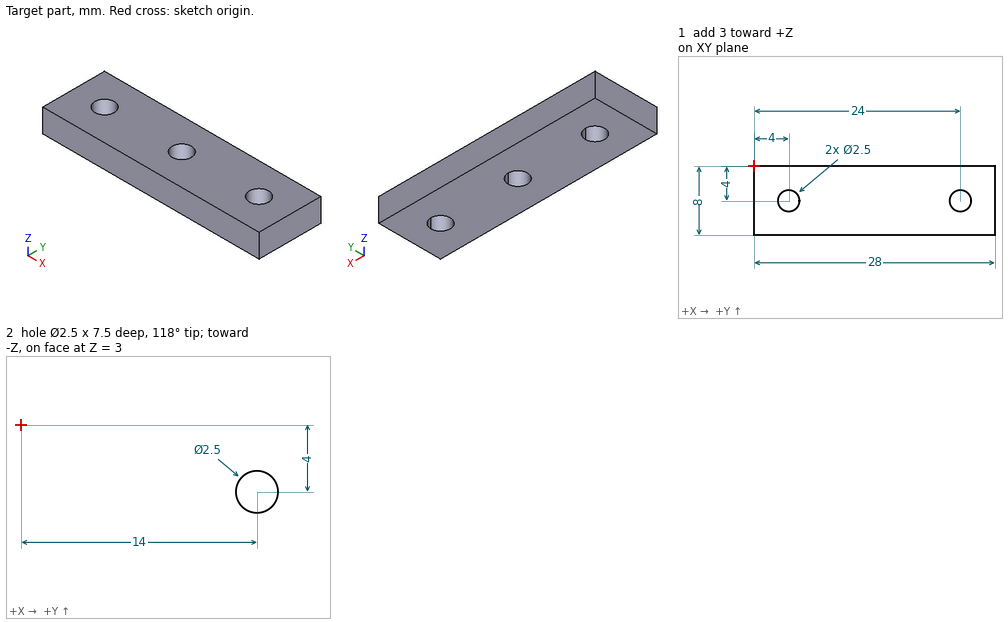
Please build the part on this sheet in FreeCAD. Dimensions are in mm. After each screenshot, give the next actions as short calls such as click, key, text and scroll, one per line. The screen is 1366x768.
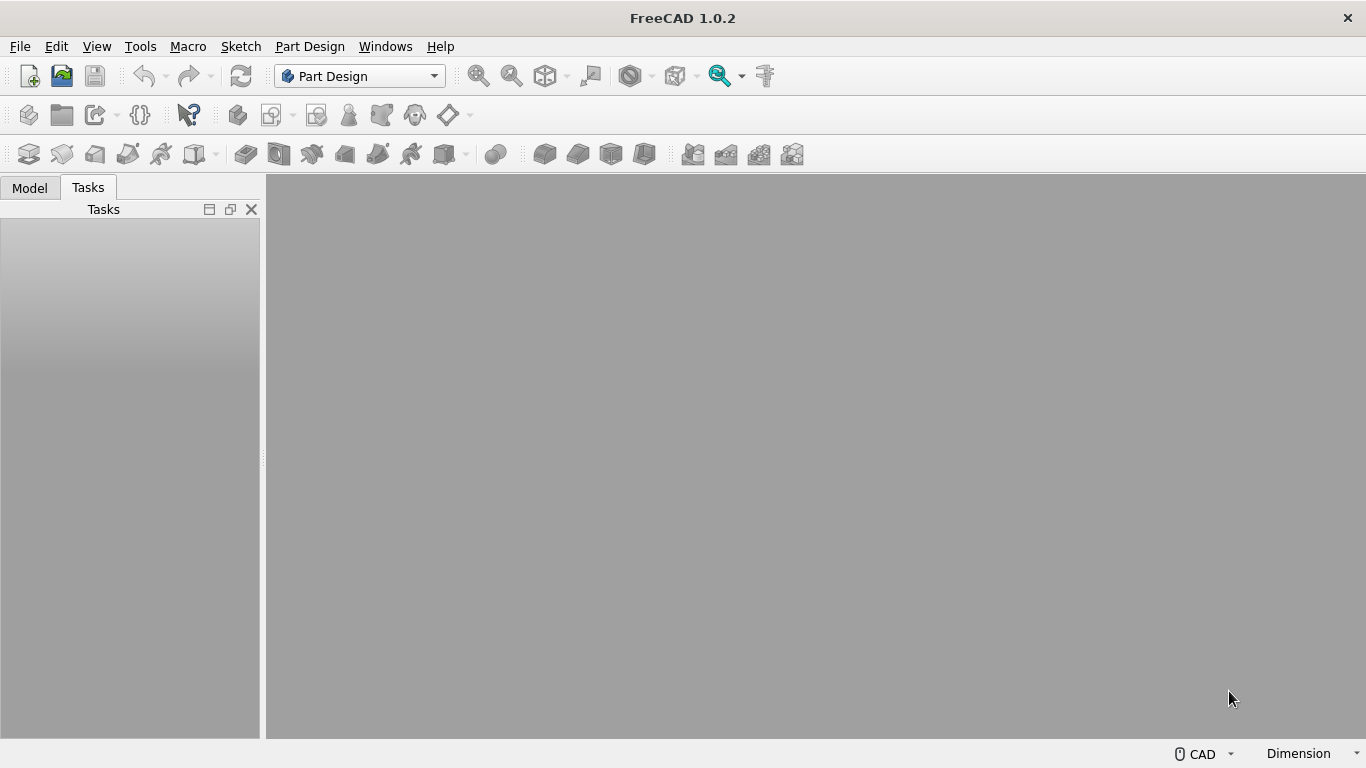
click(29, 76)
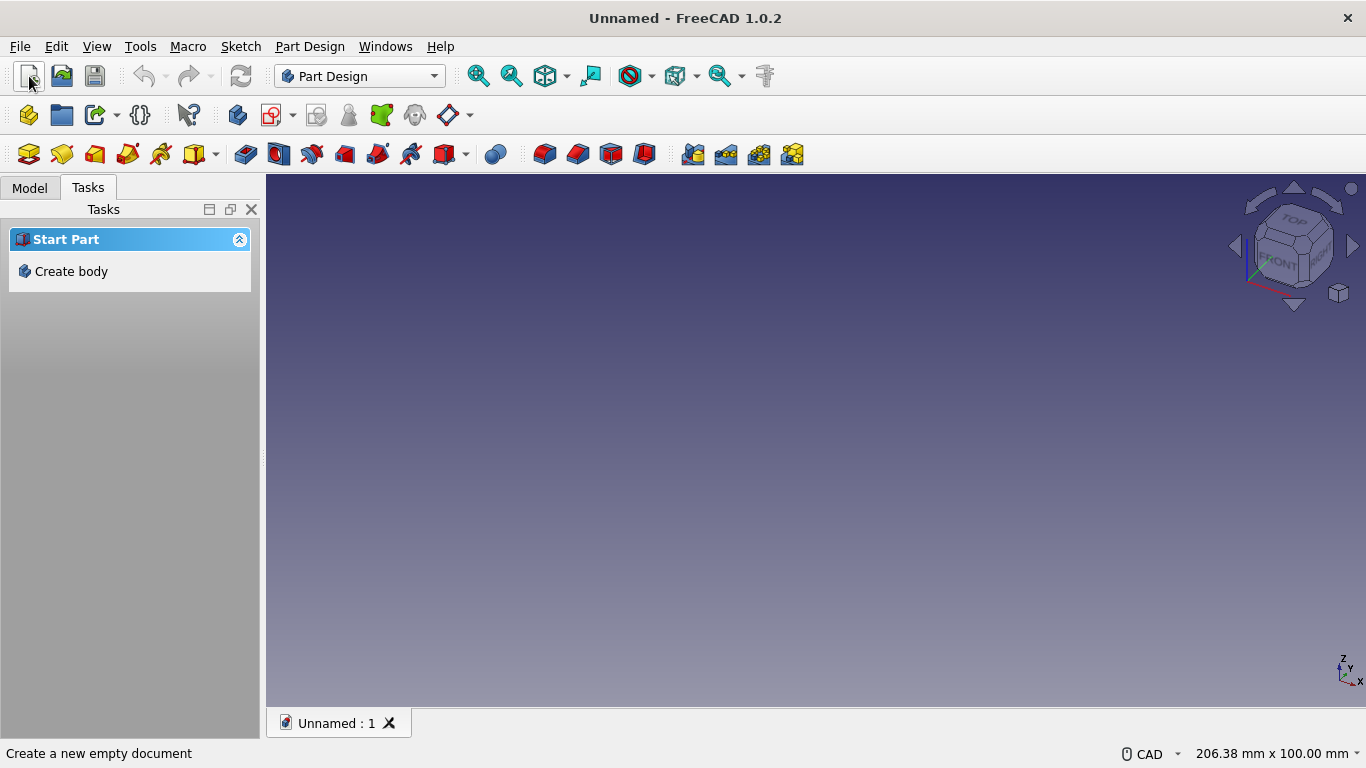
click(270, 116)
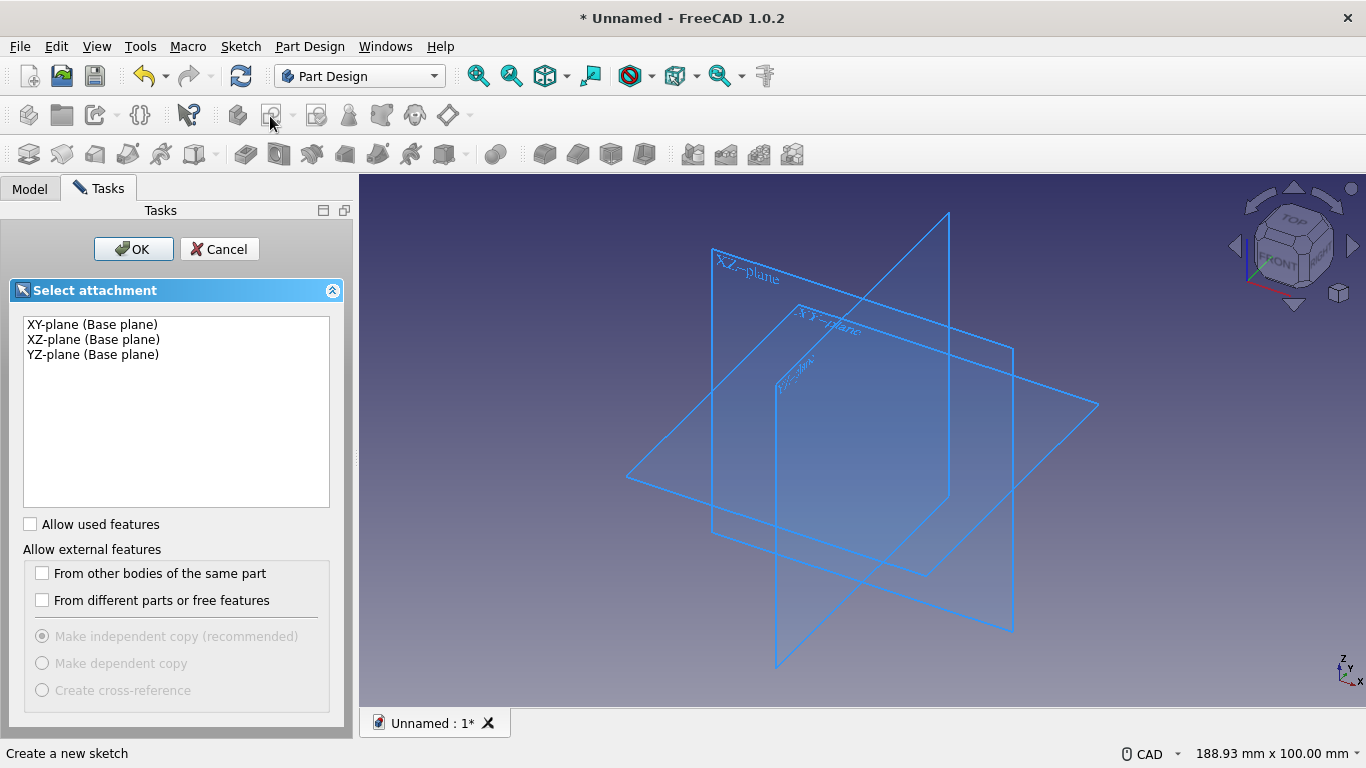
click(84, 324)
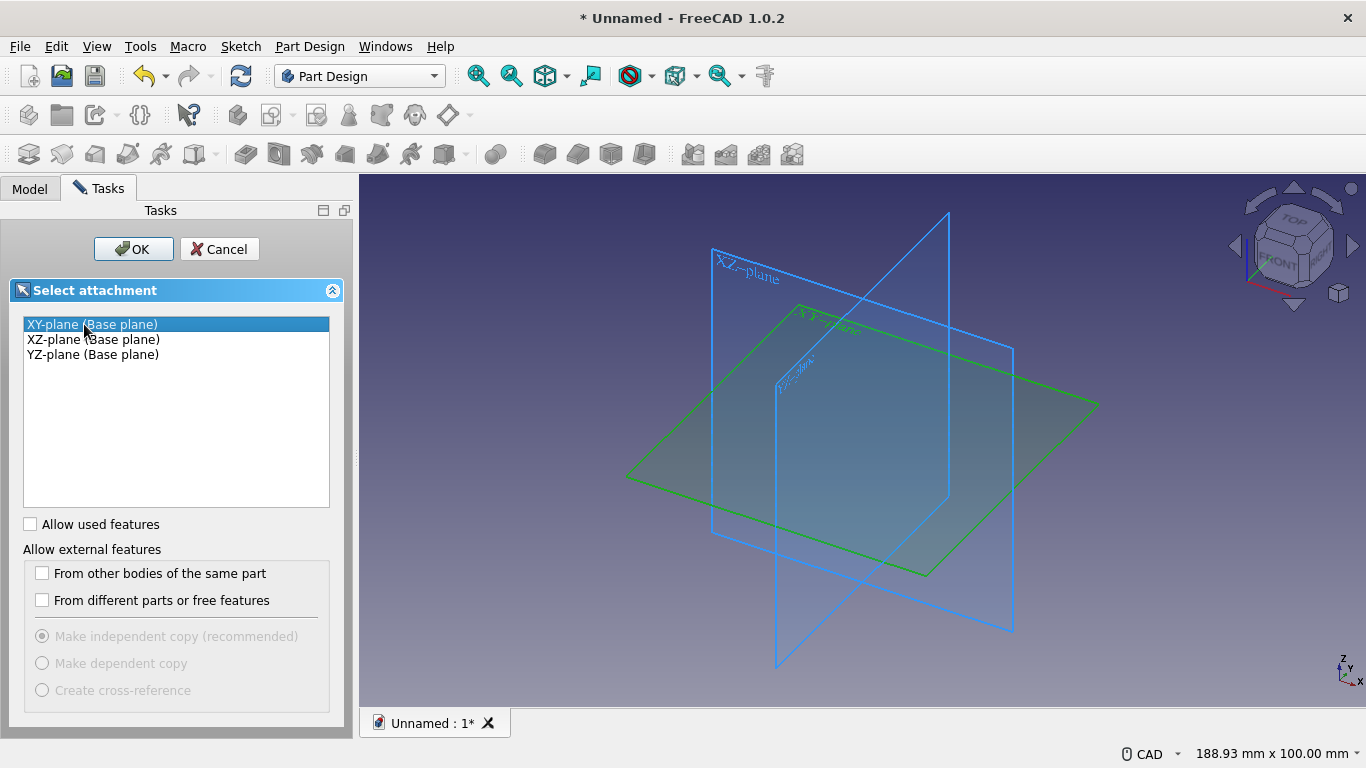
click(134, 249)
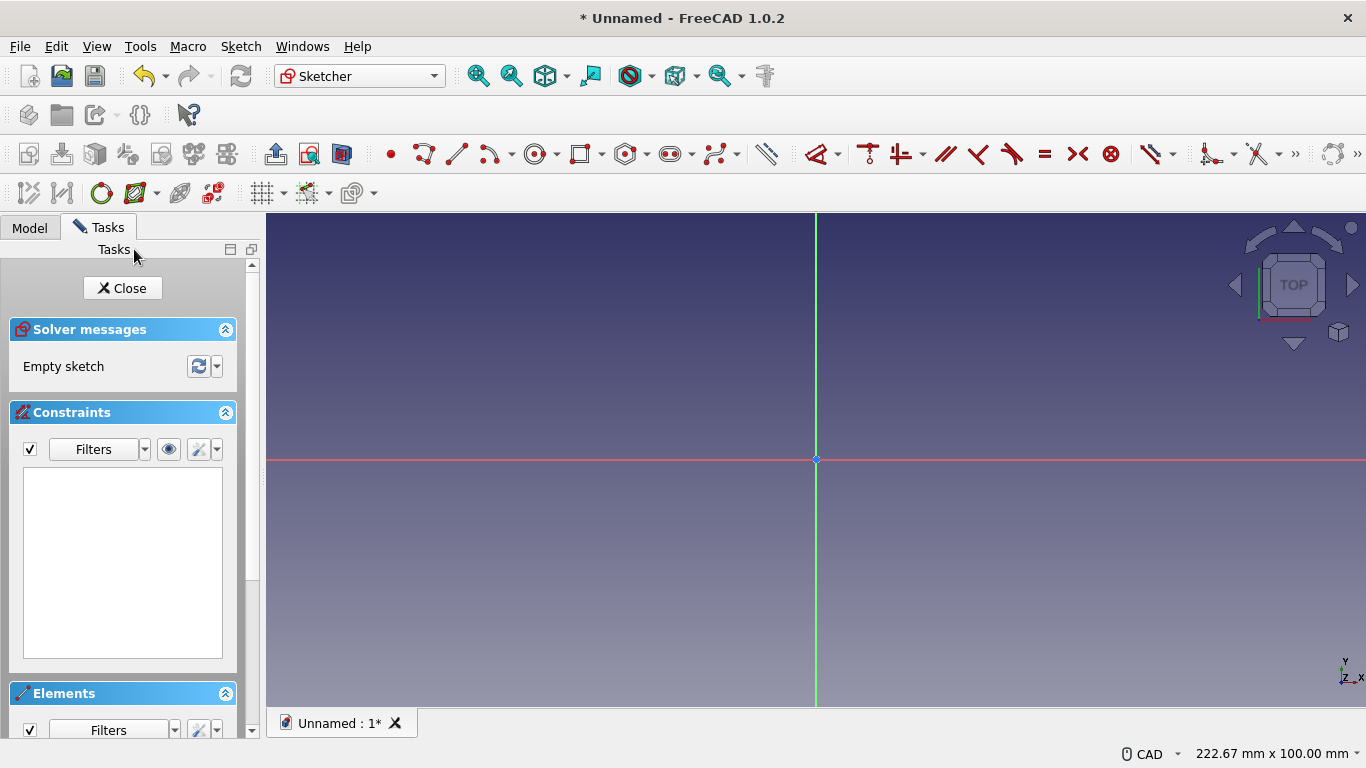
scroll(920, 485, up, 8)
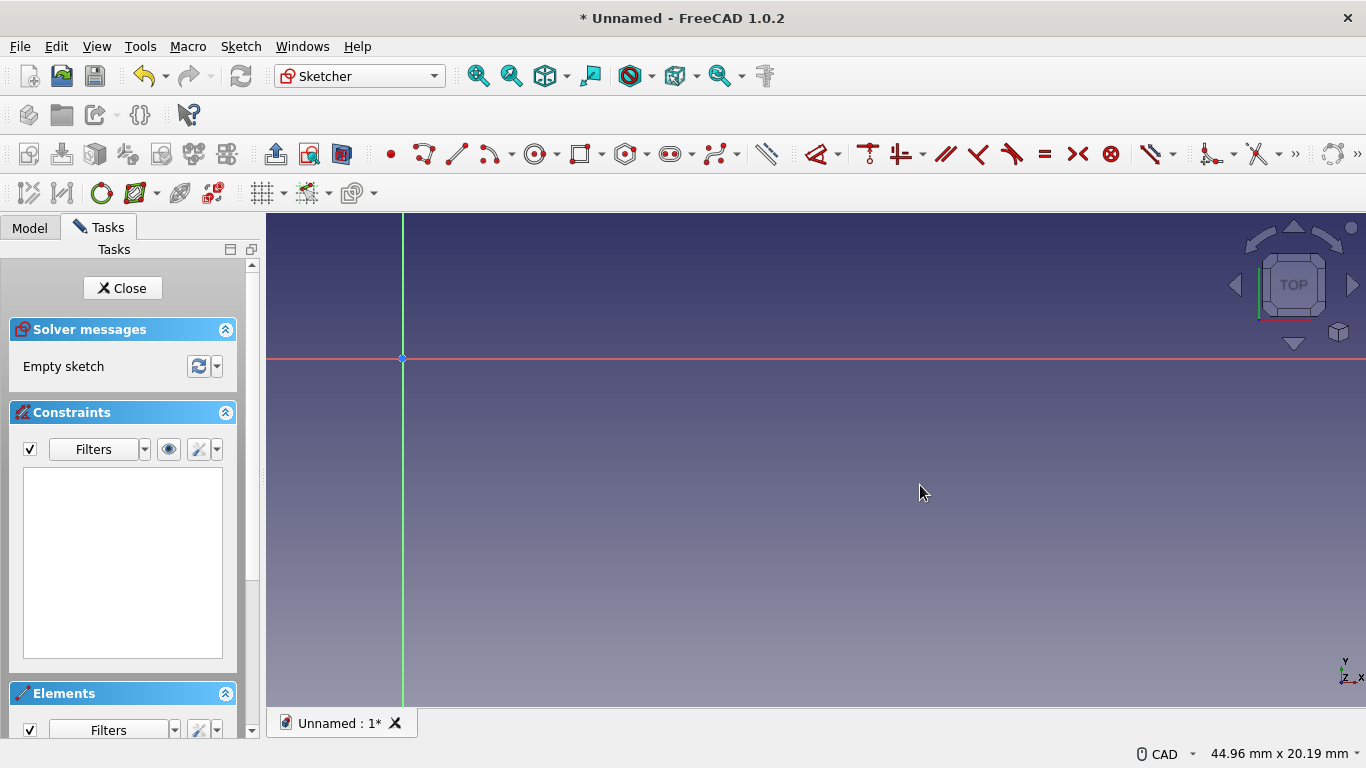
click(580, 154)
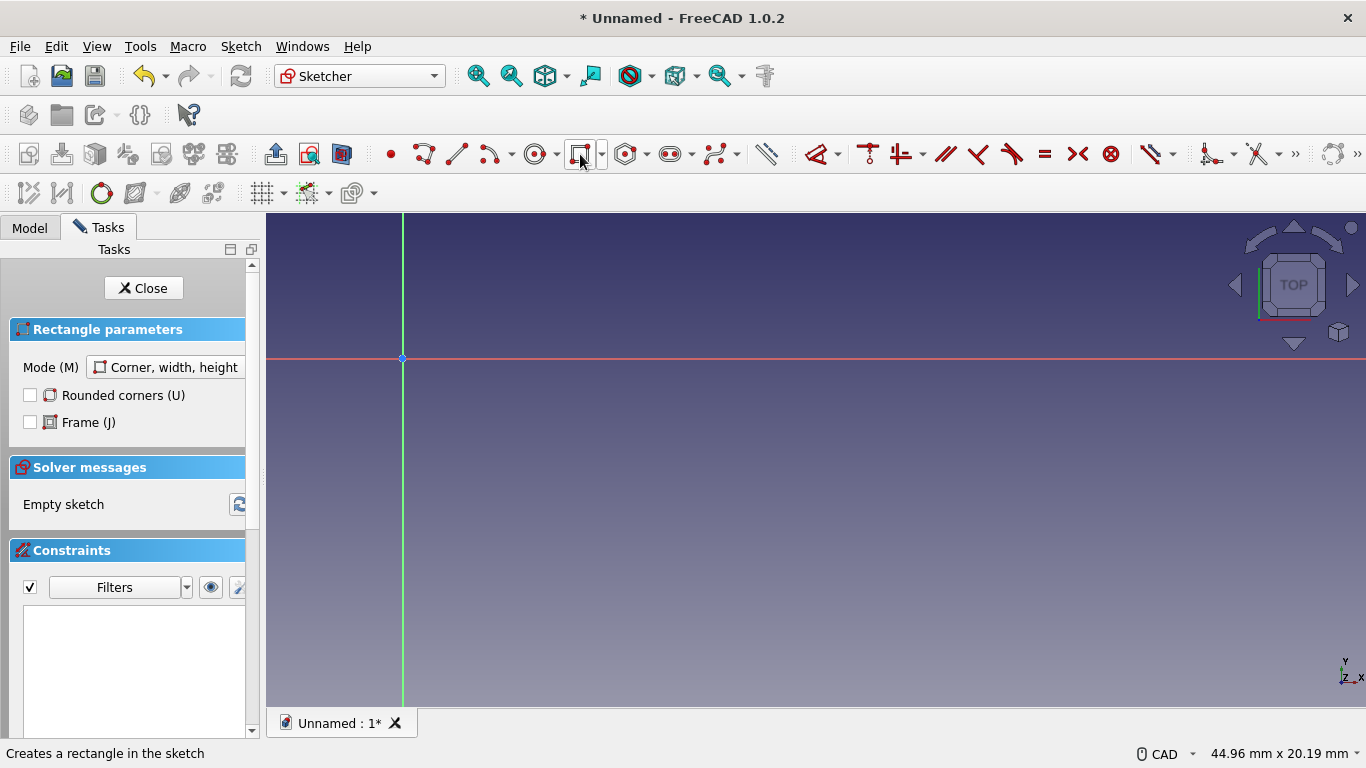
click(403, 359)
click(1088, 555)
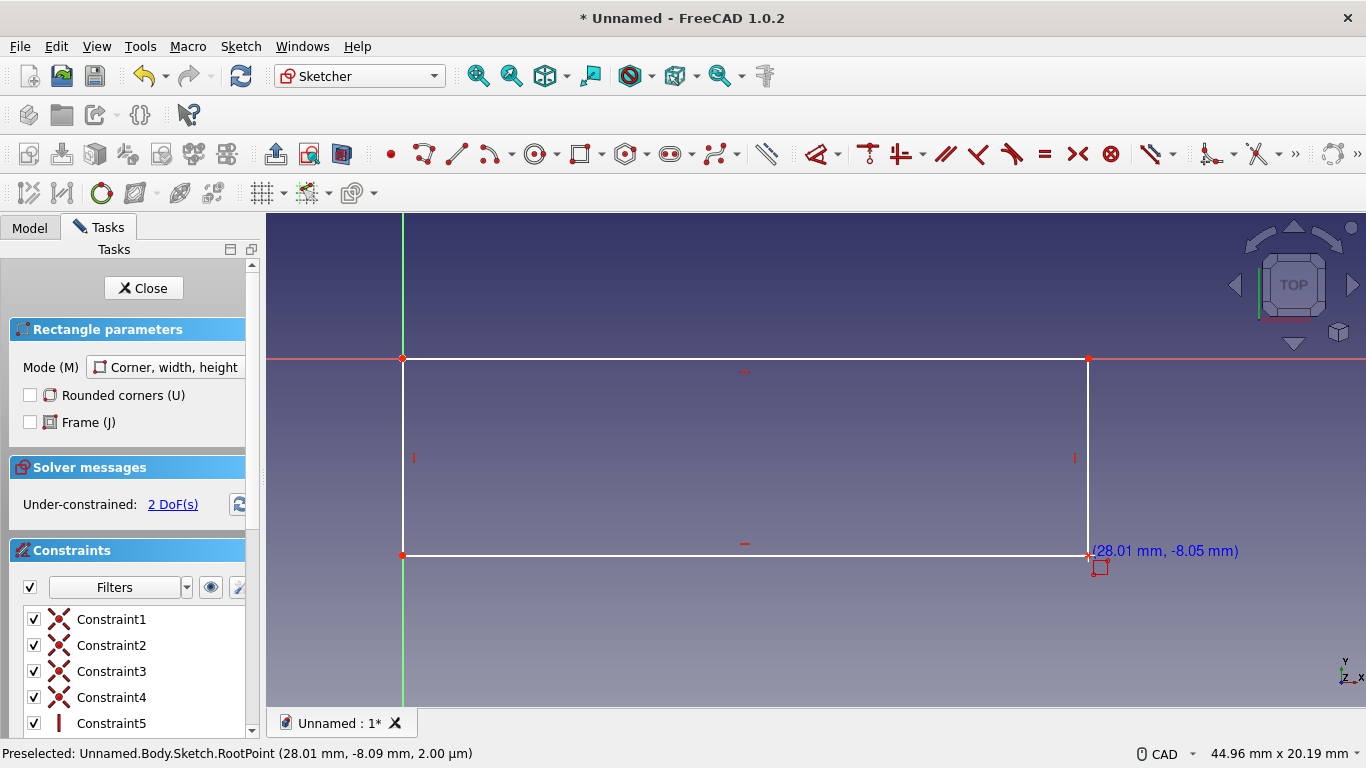
click(534, 154)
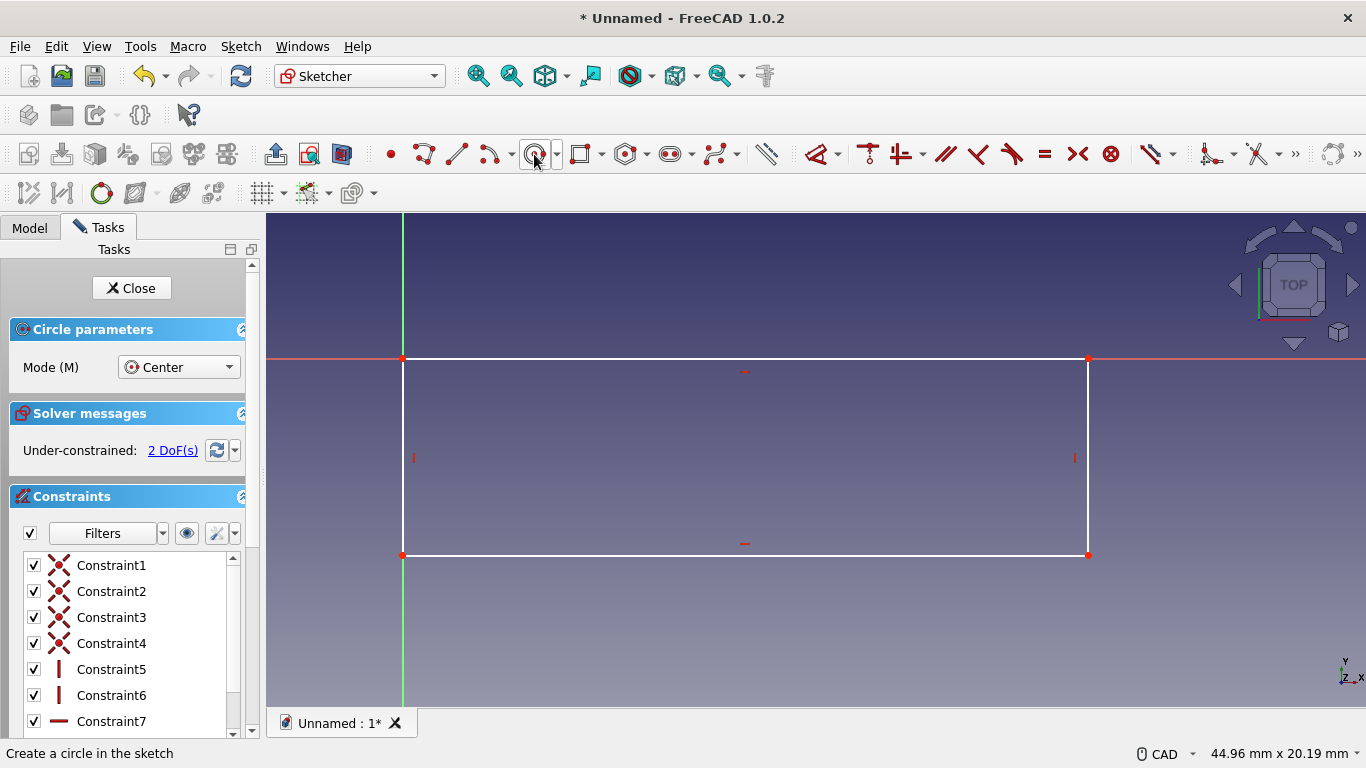
click(500, 457)
click(522, 435)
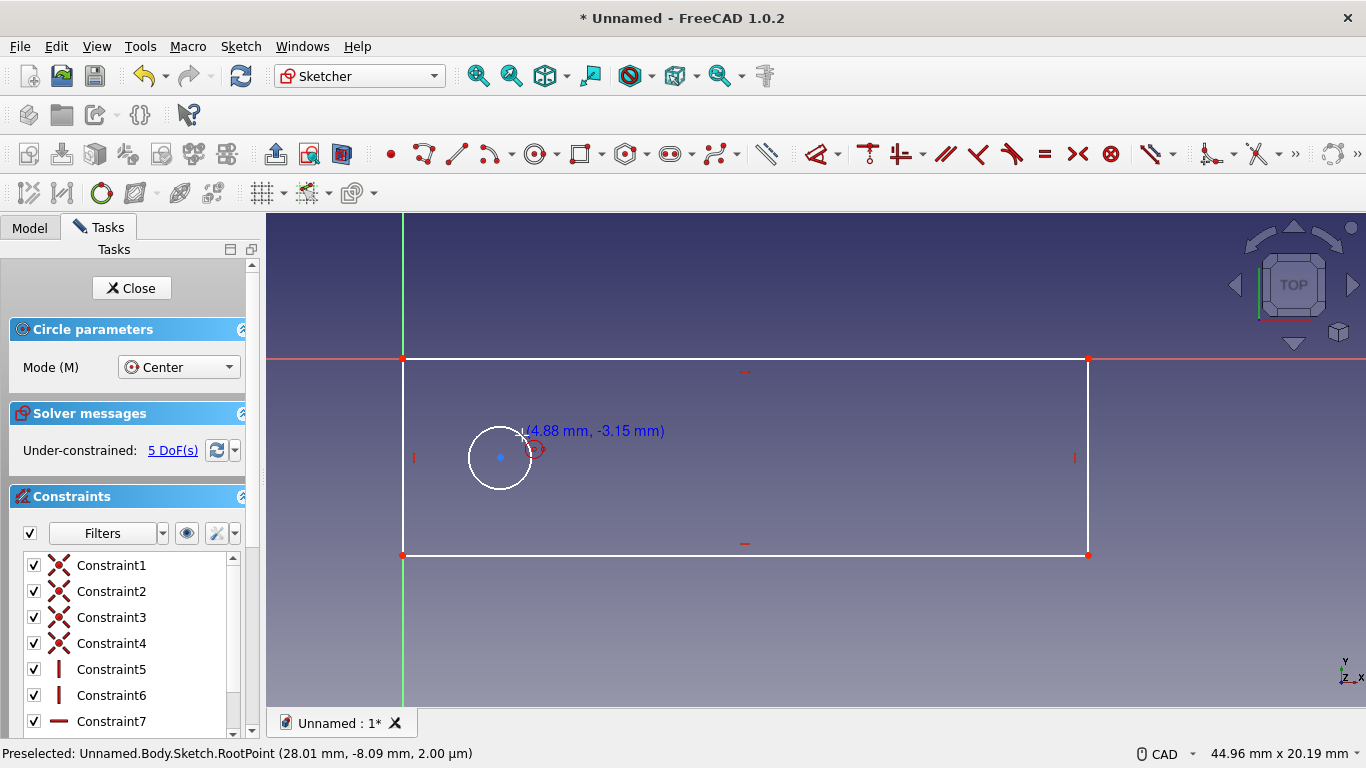
click(990, 457)
click(1011, 435)
key(Escape)